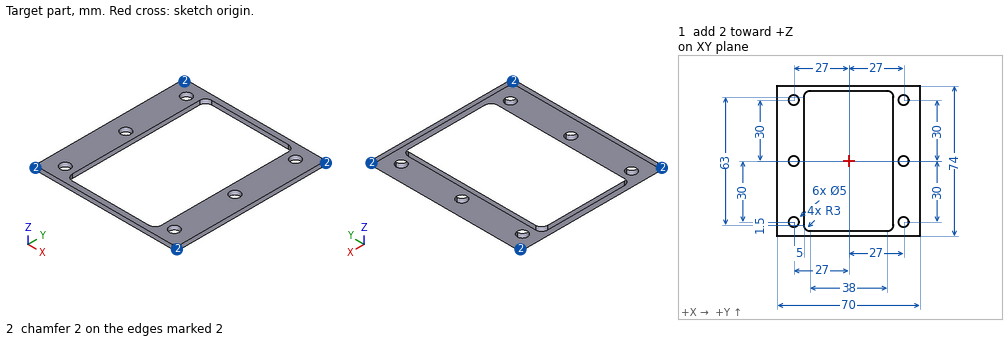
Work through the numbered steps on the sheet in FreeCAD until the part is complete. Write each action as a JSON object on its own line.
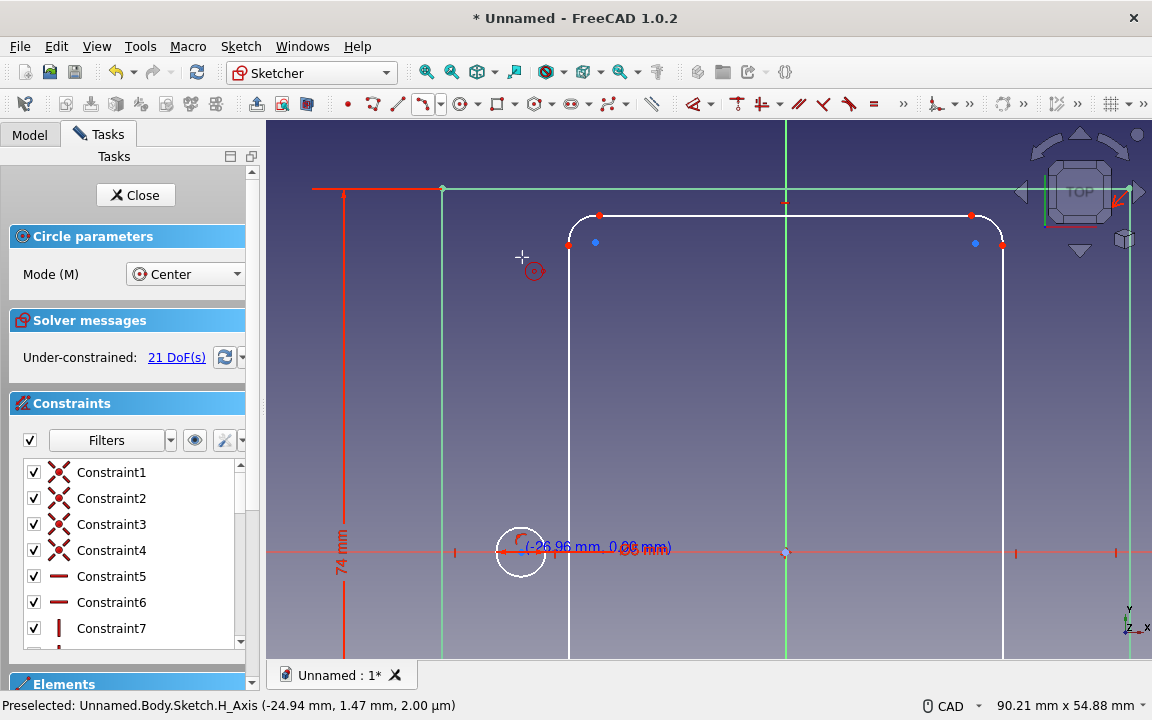
{"action": "left_click", "coordinate": [521, 257]}
{"action": "mouse_move", "coordinate": [538, 240]}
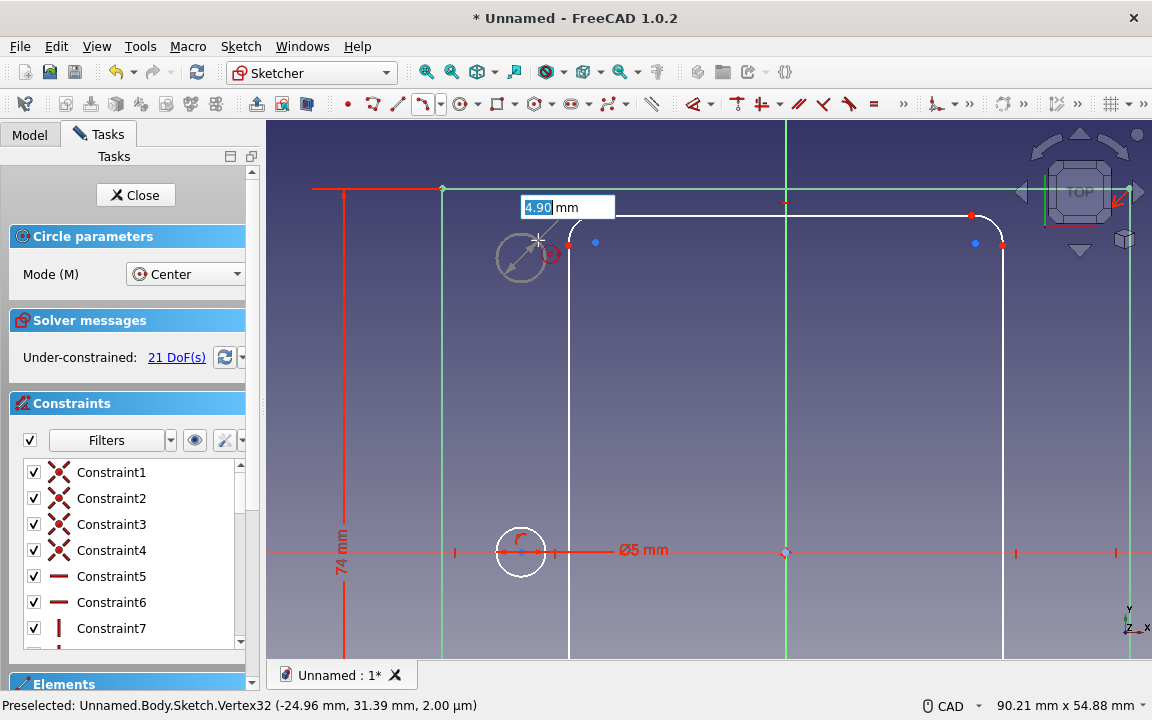
{"action": "type", "text": "5"}
{"action": "key", "text": "Return"}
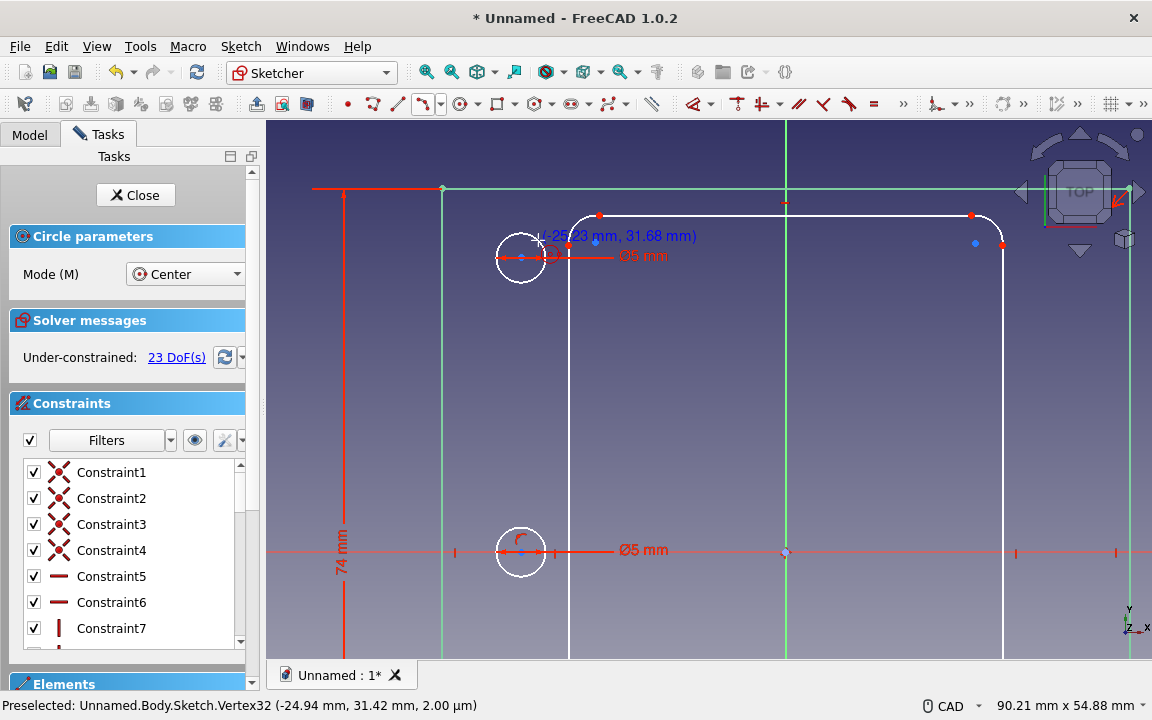
{"action": "scroll", "coordinate": [522, 257], "scroll_direction": "down", "scroll_amount": 4}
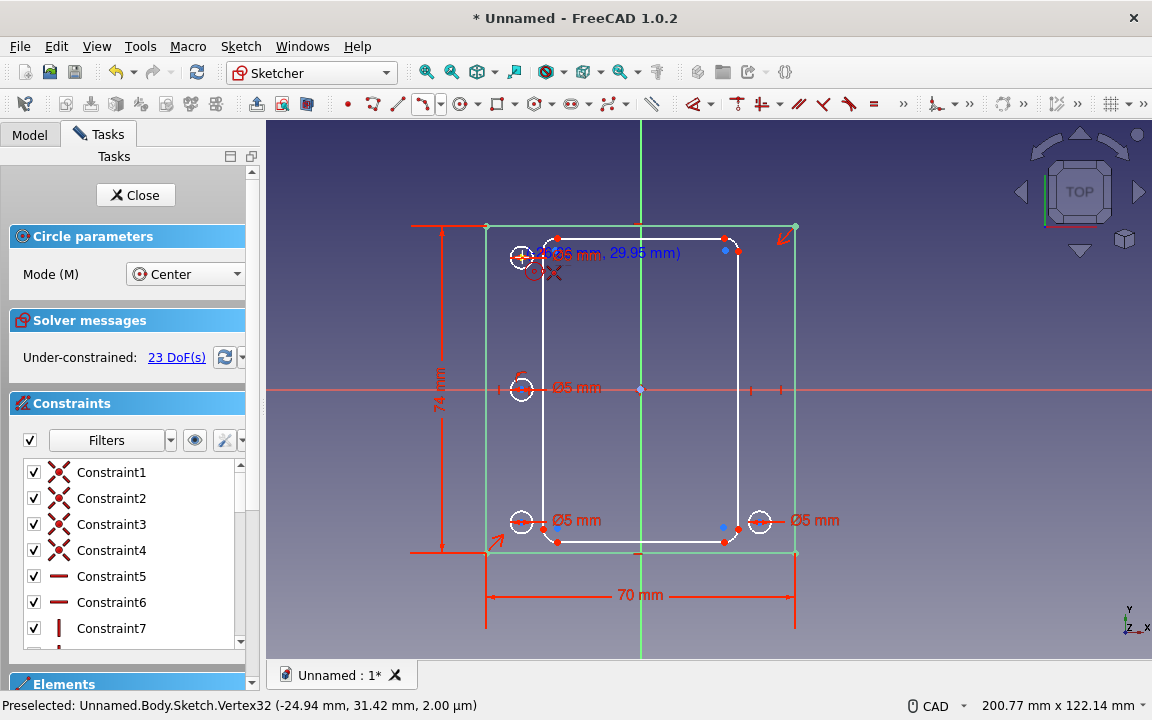
{"action": "scroll", "coordinate": [760, 390], "scroll_direction": "up", "scroll_amount": 4}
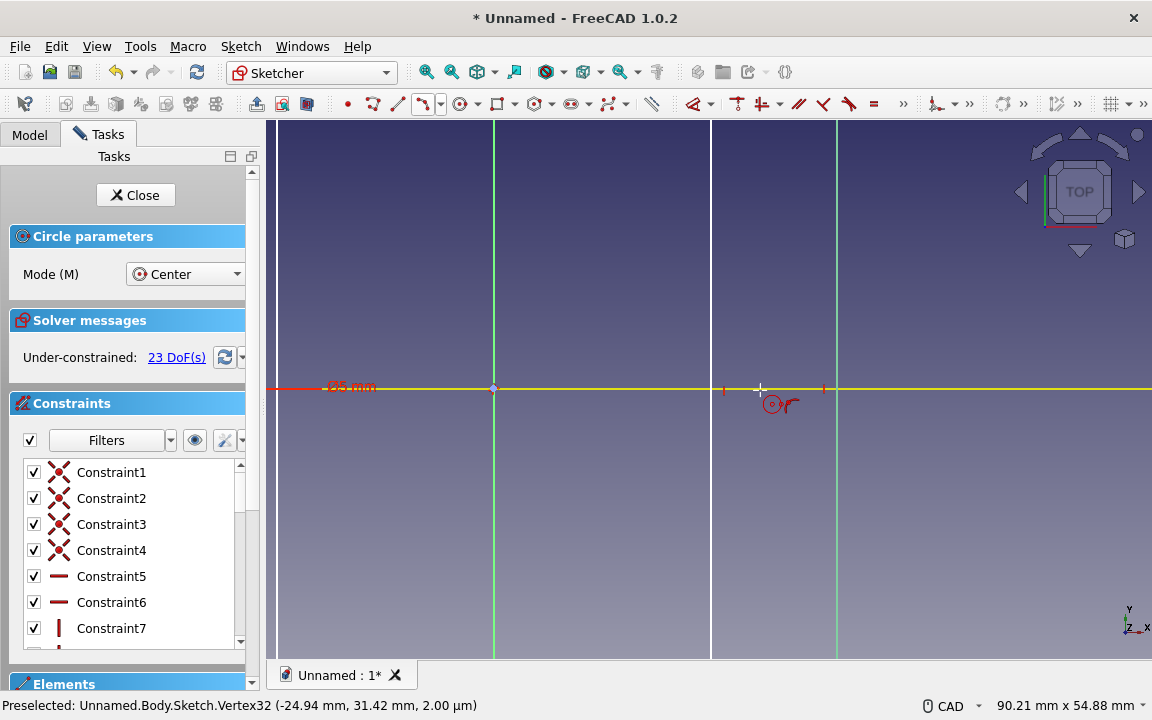
{"action": "left_click", "coordinate": [759, 389]}
{"action": "mouse_move", "coordinate": [776, 371]}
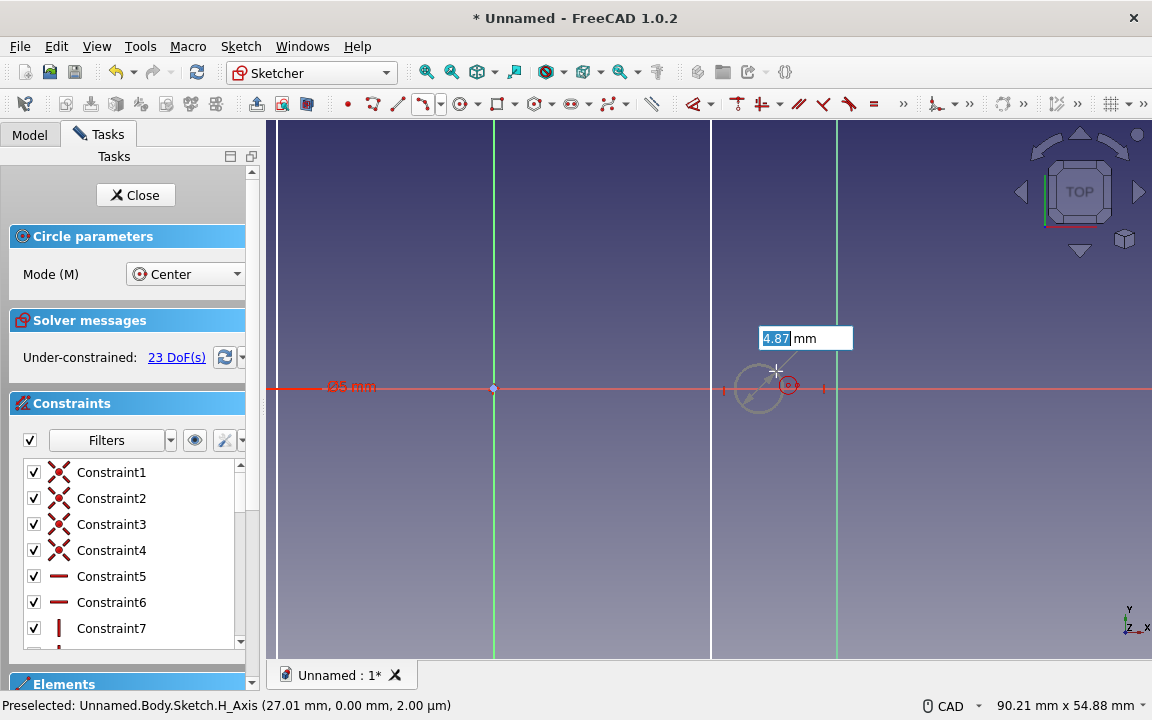
{"action": "type", "text": "5"}
{"action": "key", "text": "Return"}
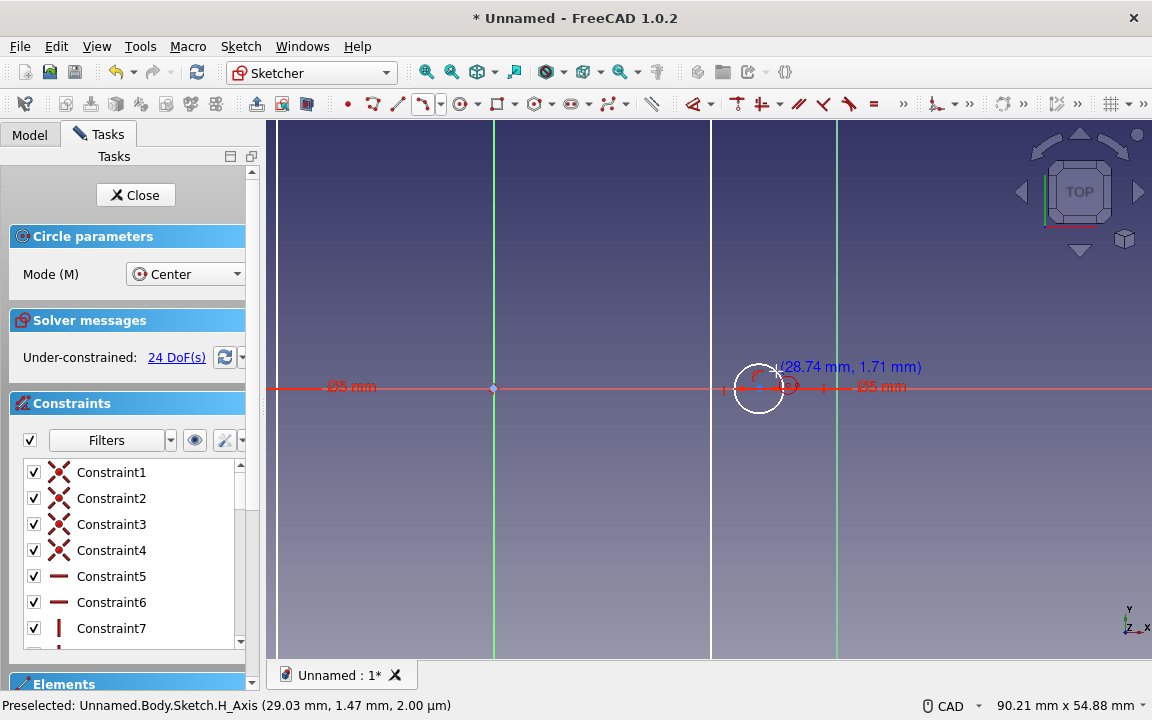
{"action": "scroll", "coordinate": [760, 390], "scroll_direction": "down", "scroll_amount": 4}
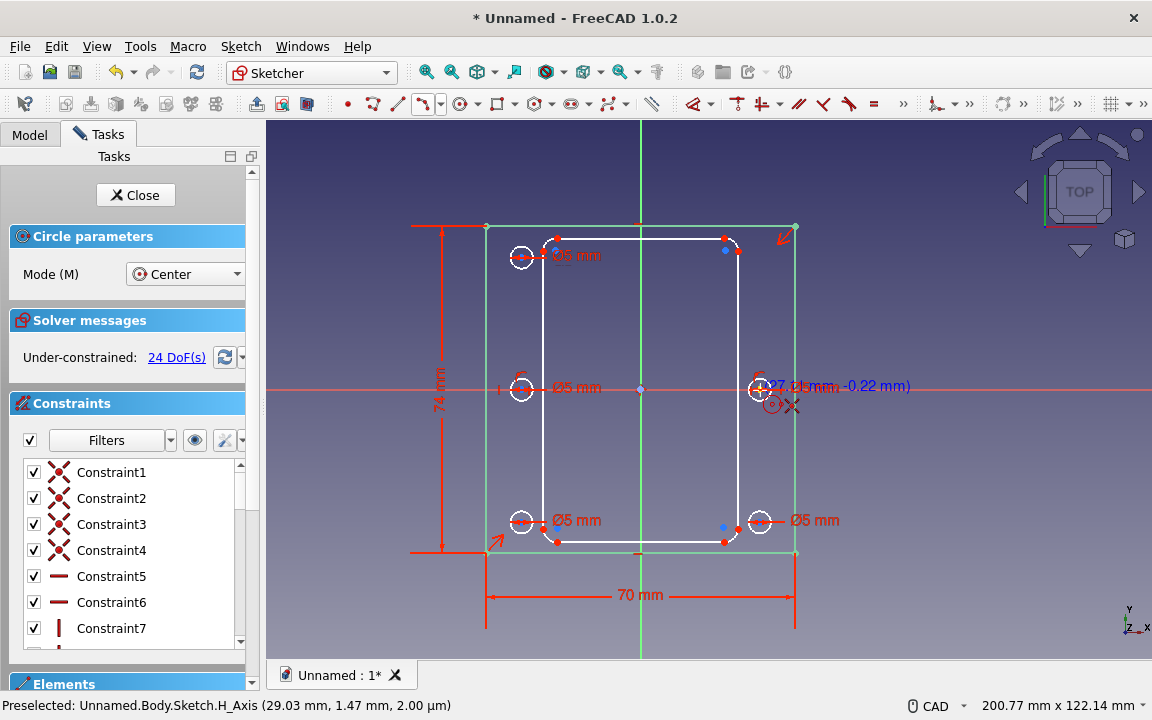
{"action": "scroll", "coordinate": [760, 257], "scroll_direction": "up", "scroll_amount": 4}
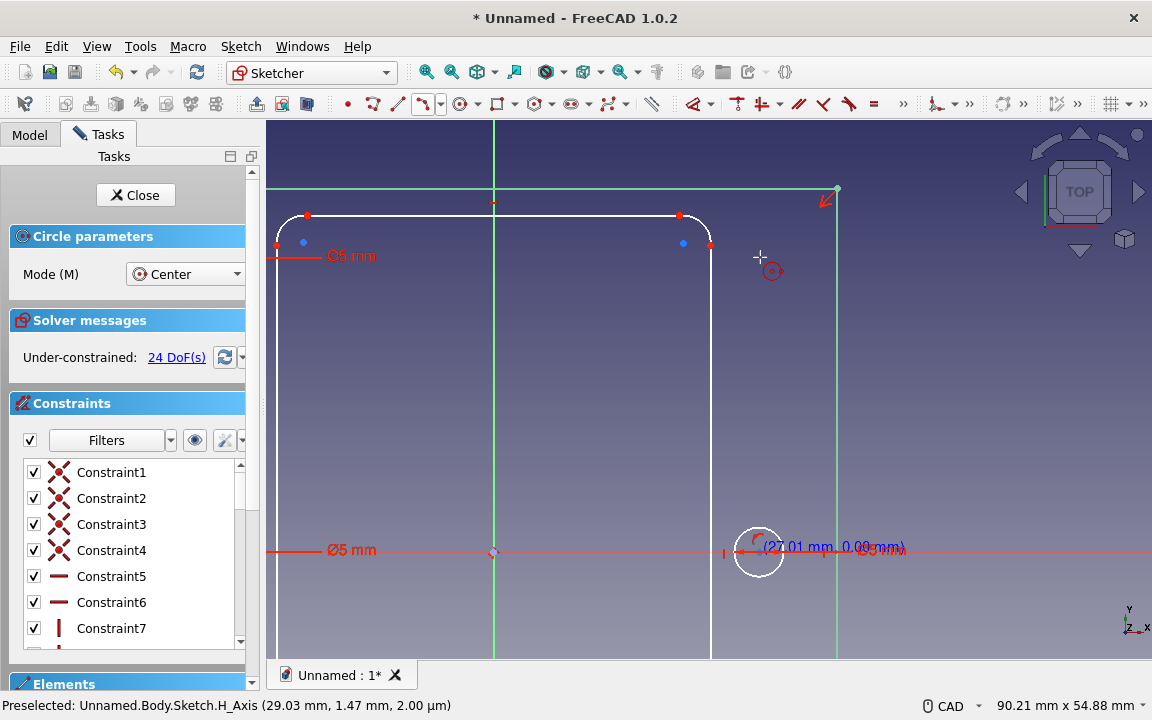
{"action": "left_click", "coordinate": [759, 257]}
{"action": "mouse_move", "coordinate": [776, 240]}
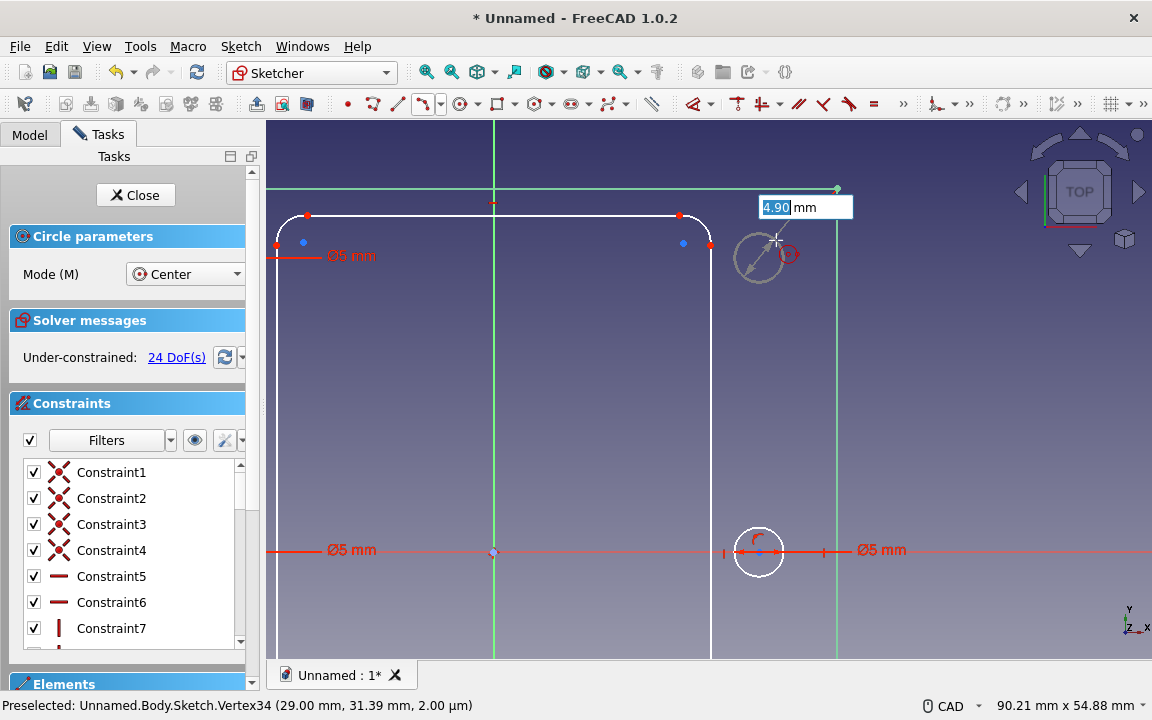
{"action": "type", "text": "5"}
{"action": "key", "text": "Return"}
{"action": "key", "text": "Escape"}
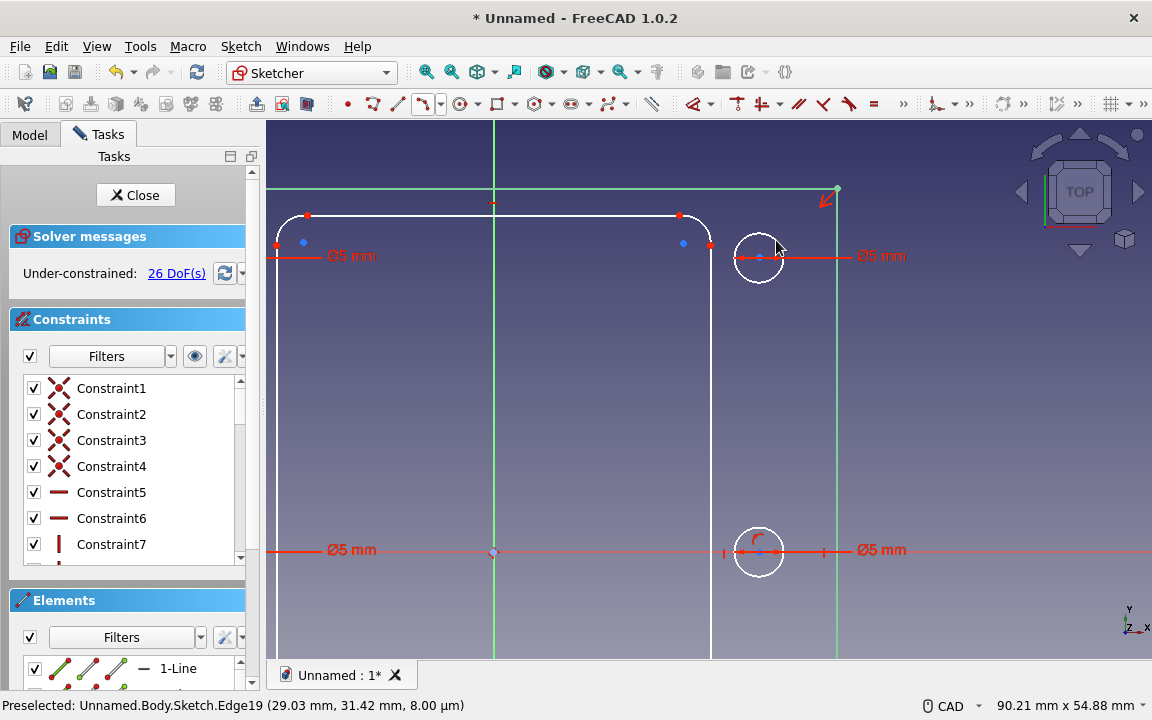
{"action": "scroll", "coordinate": [760, 257], "scroll_direction": "down", "scroll_amount": 4}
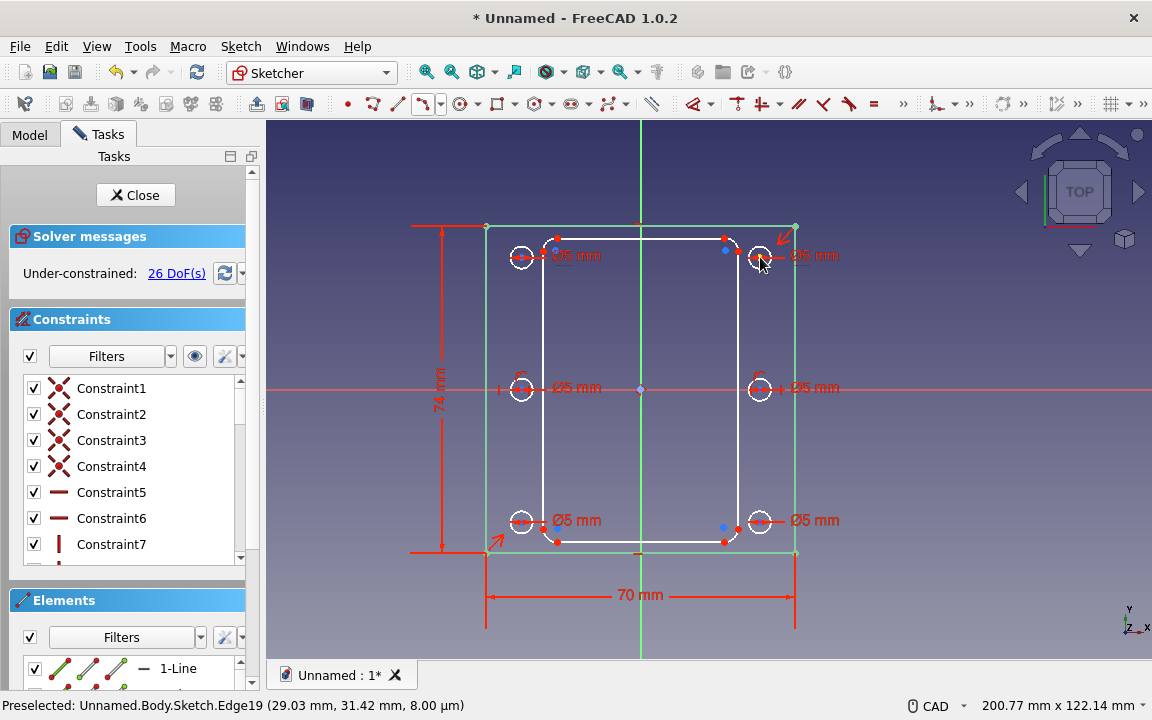
{"action": "scroll", "coordinate": [674, 542], "scroll_direction": "up", "scroll_amount": 2}